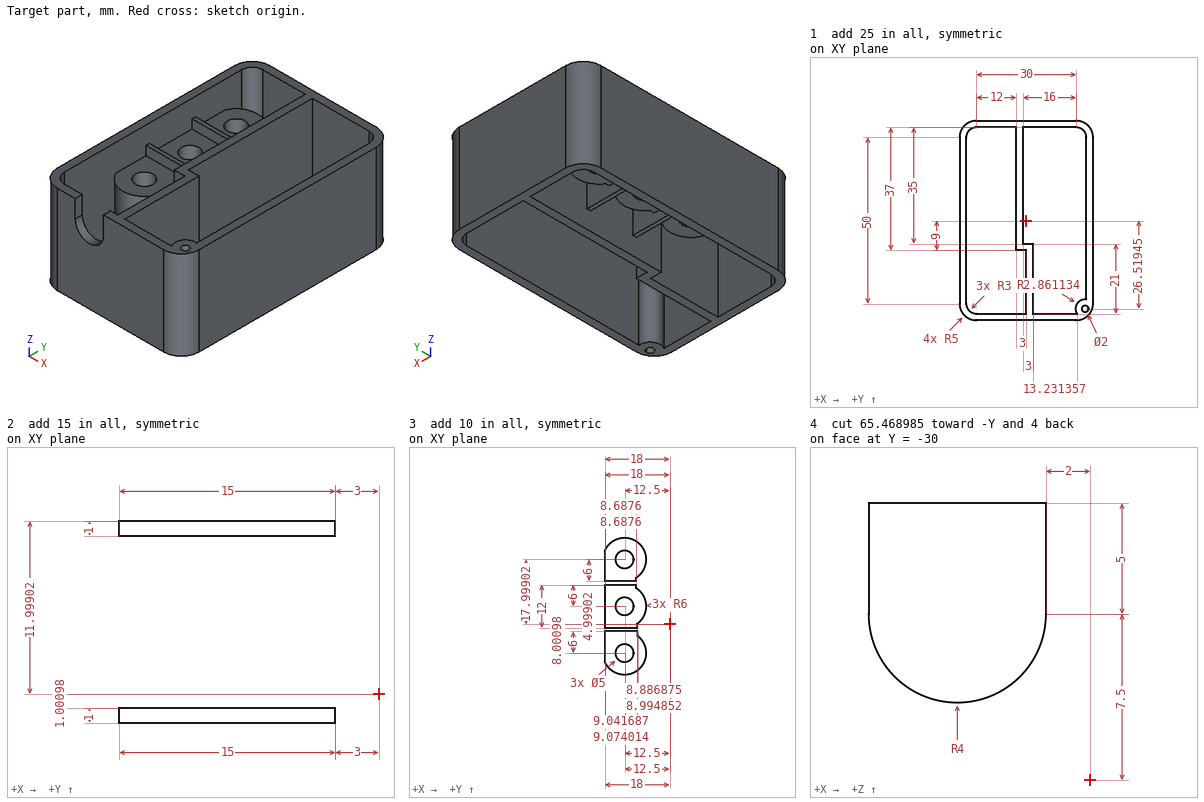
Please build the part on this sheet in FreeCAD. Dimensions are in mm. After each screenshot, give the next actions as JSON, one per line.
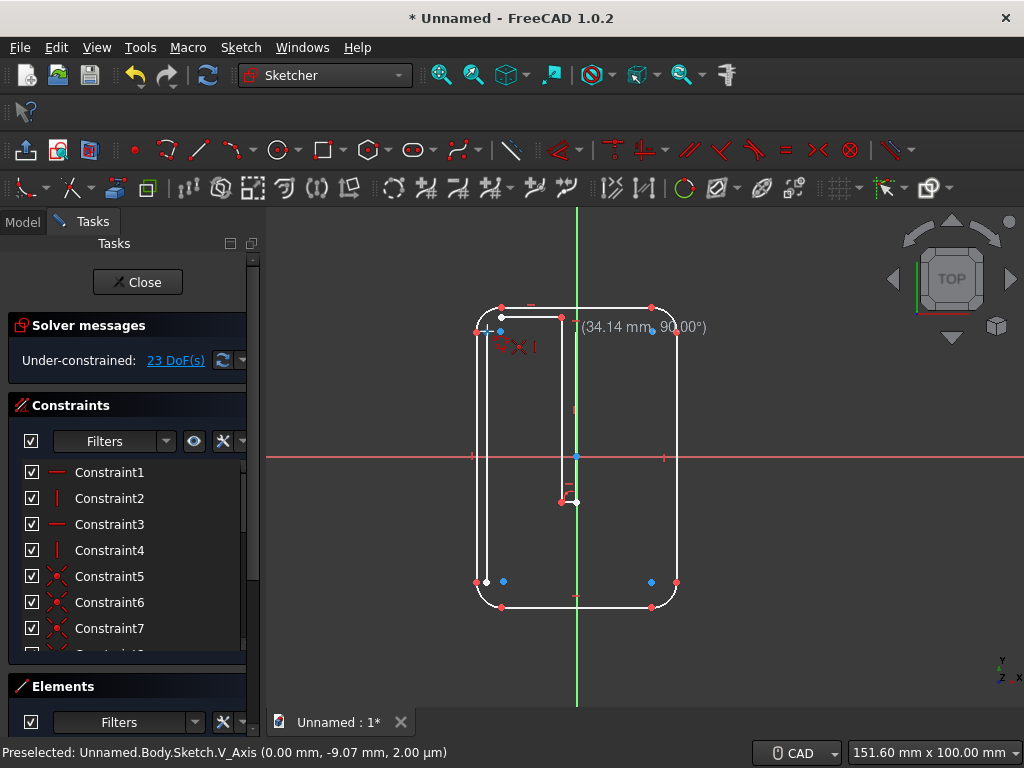
{"action": "scroll", "coordinate": [577, 597], "scroll_direction": "up", "scroll_amount": 3}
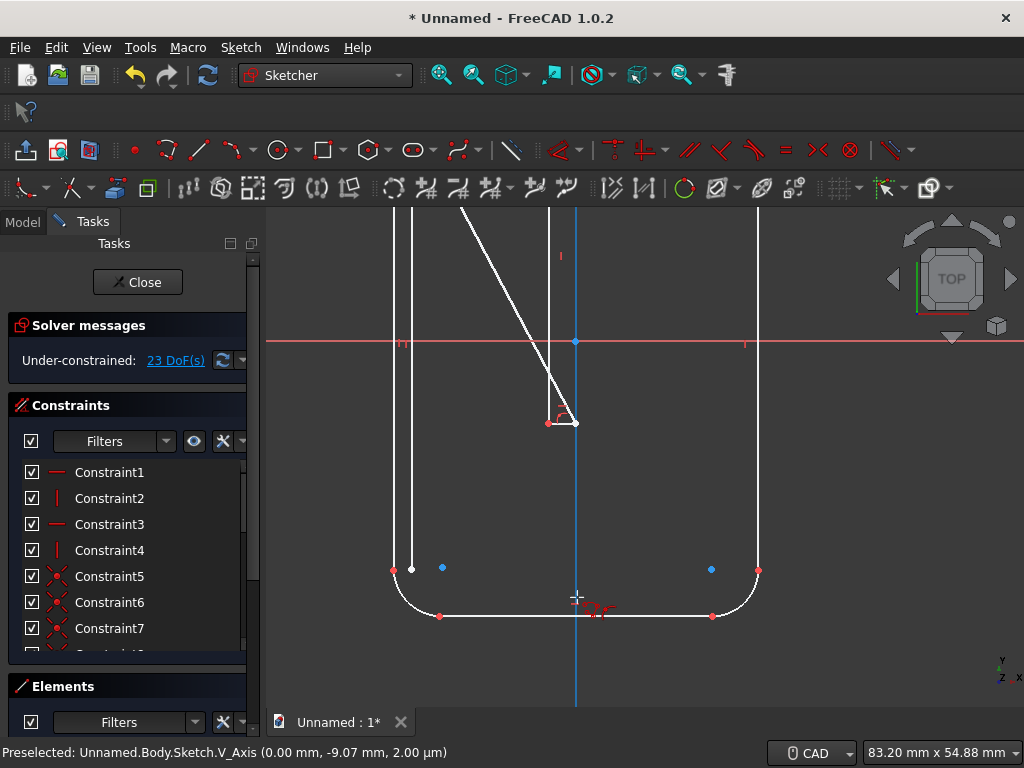
{"action": "left_click", "coordinate": [585, 596]}
{"action": "left_click", "coordinate": [439, 596]}
{"action": "right_click", "coordinate": [439, 596]}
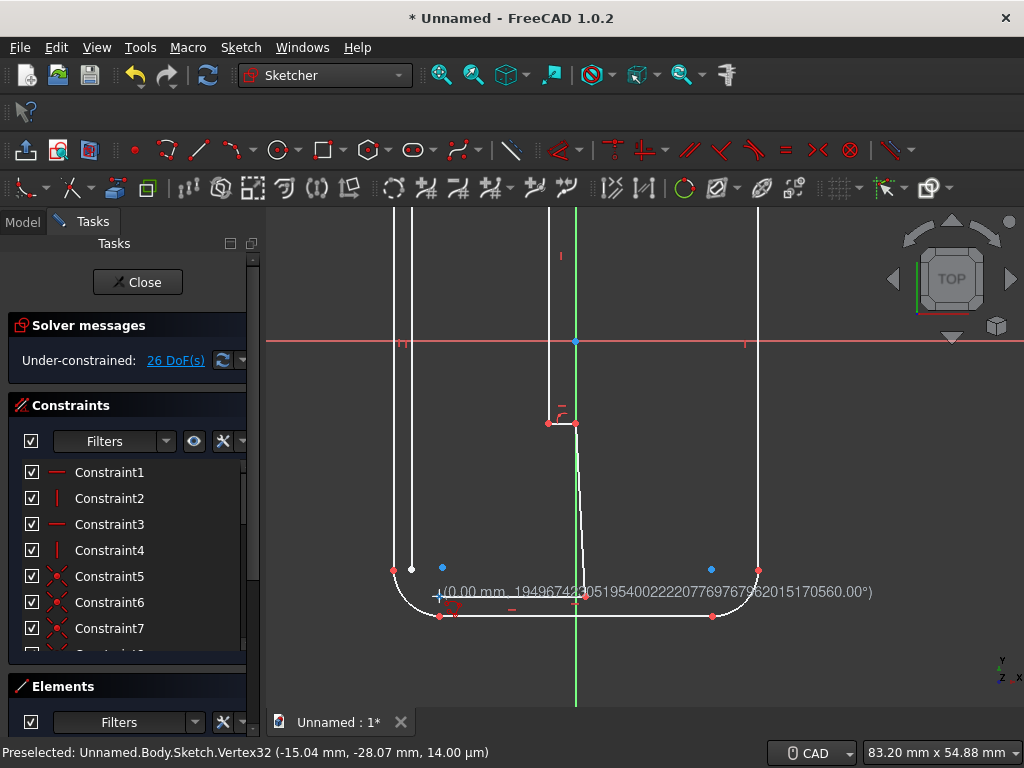
{"action": "left_click", "coordinate": [232, 150]}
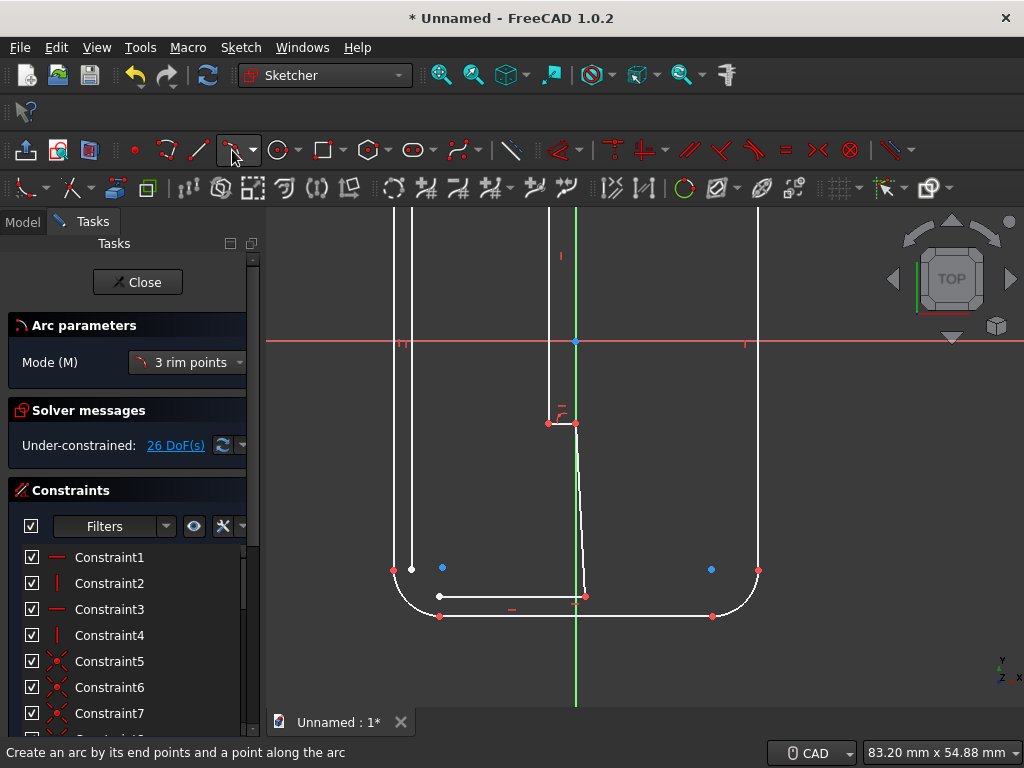
{"action": "scroll", "coordinate": [577, 598], "scroll_direction": "down", "scroll_amount": 3}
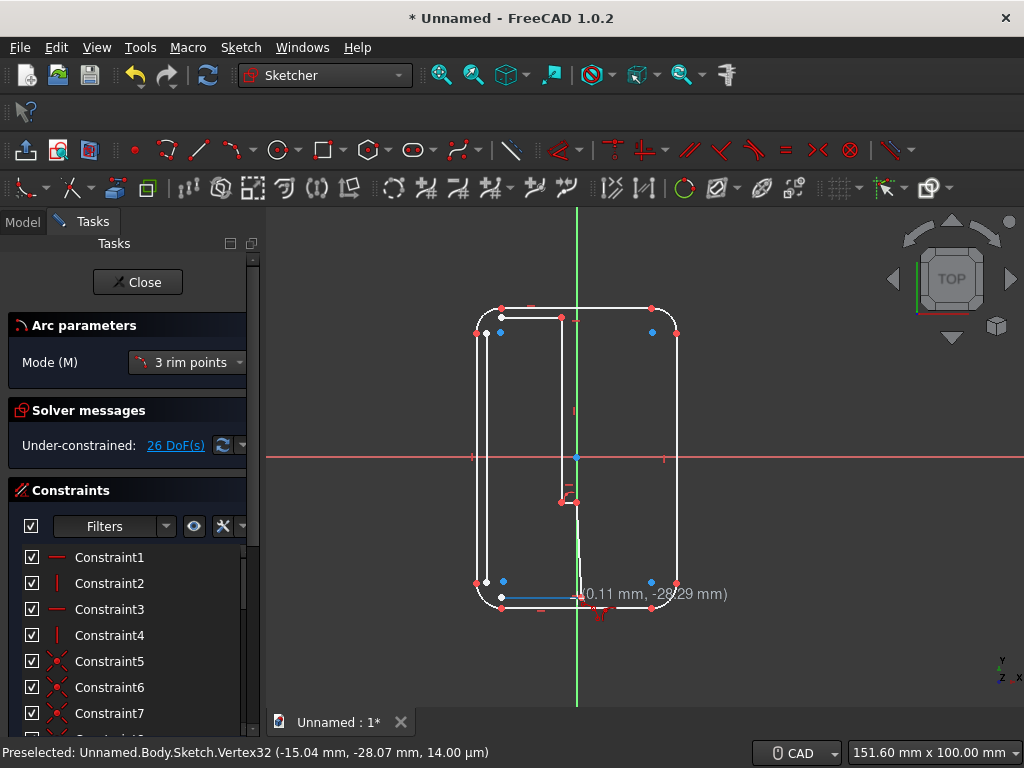
{"action": "scroll", "coordinate": [487, 332], "scroll_direction": "up", "scroll_amount": 3}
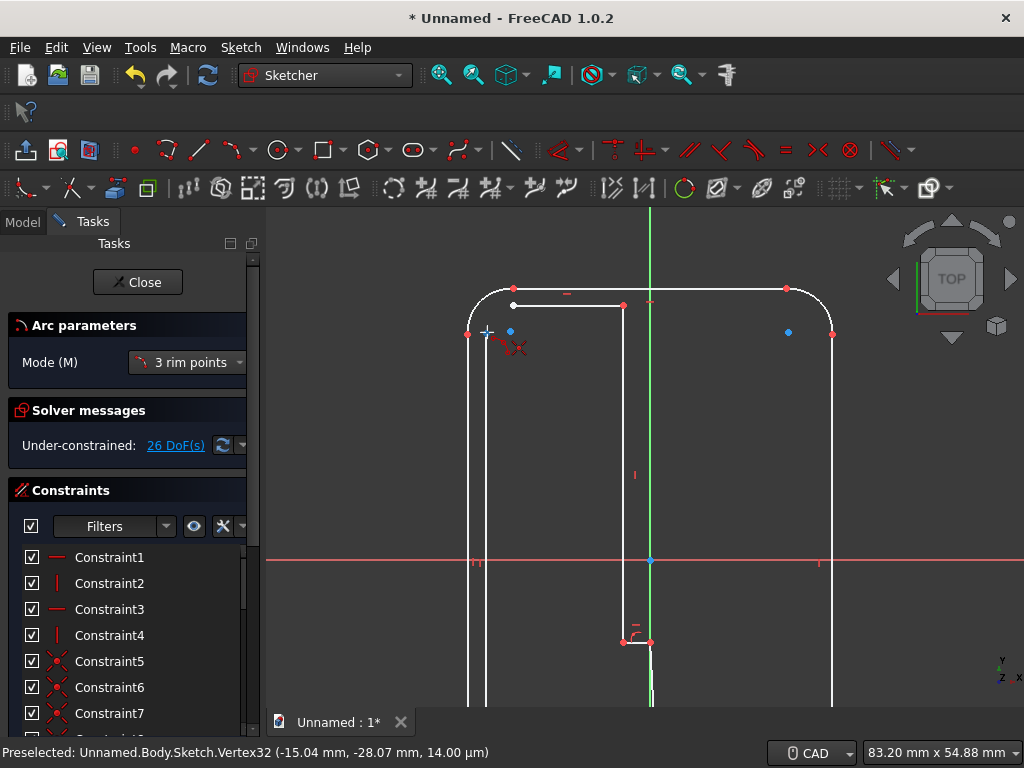
{"action": "left_click", "coordinate": [486, 334]}
{"action": "left_click", "coordinate": [513, 306]}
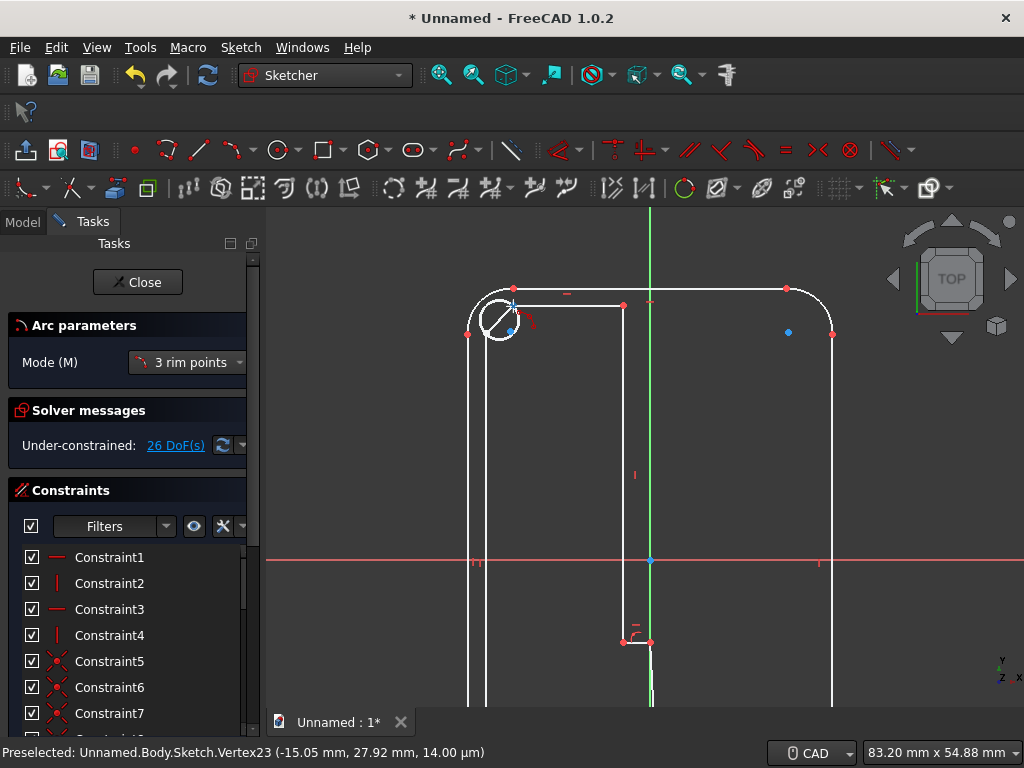
{"action": "scroll", "coordinate": [494, 313], "scroll_direction": "up", "scroll_amount": 4}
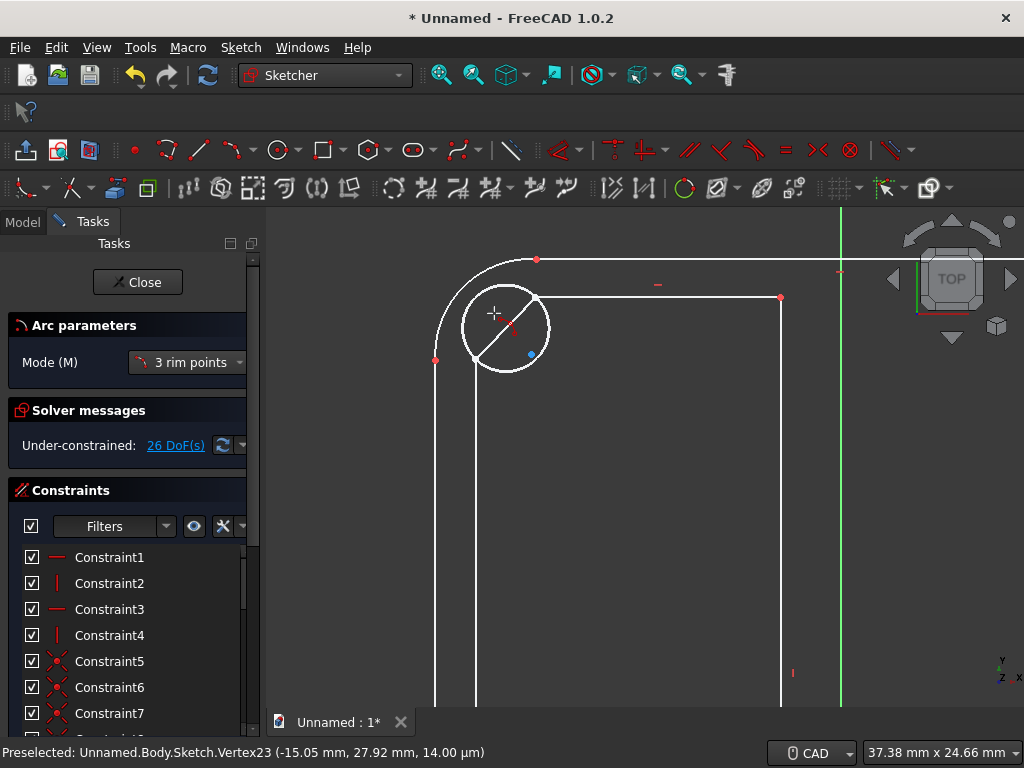
{"action": "left_click", "coordinate": [494, 313]}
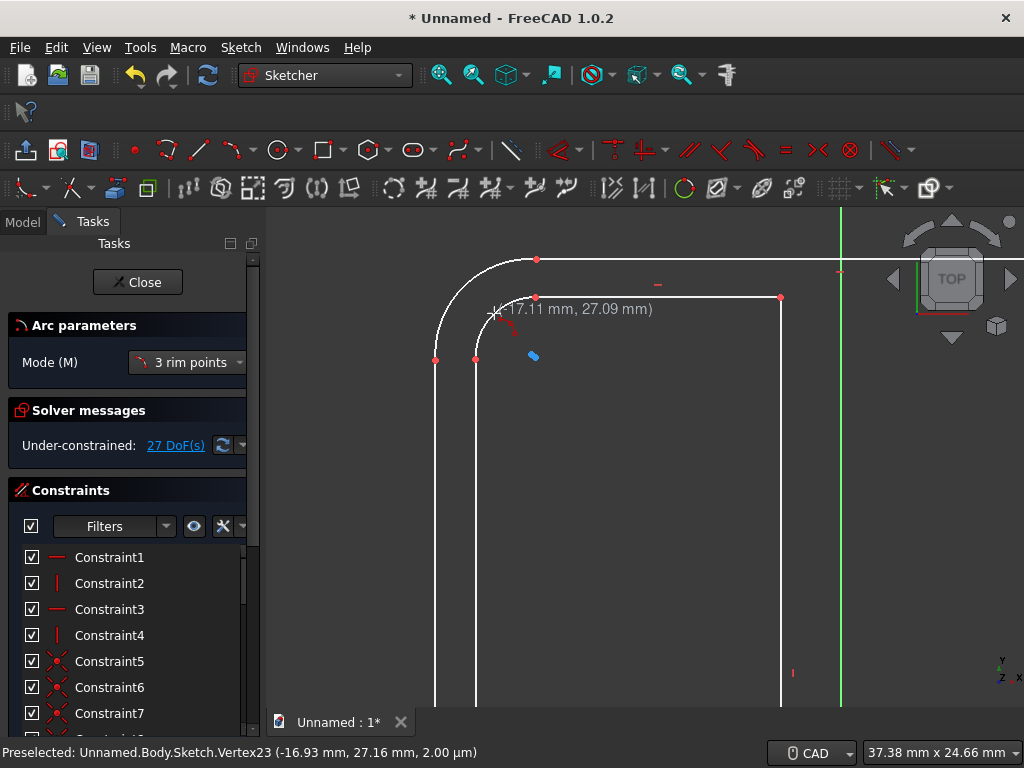
{"action": "scroll", "coordinate": [490, 324], "scroll_direction": "down", "scroll_amount": 7}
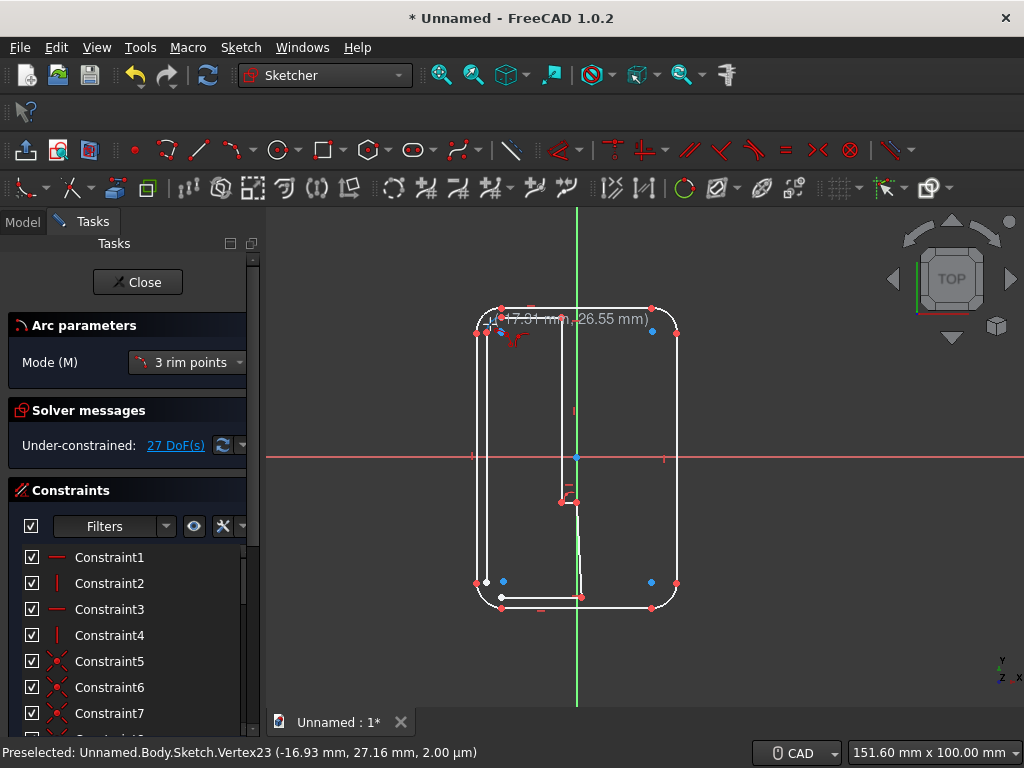
{"action": "scroll", "coordinate": [502, 597], "scroll_direction": "up", "scroll_amount": 3}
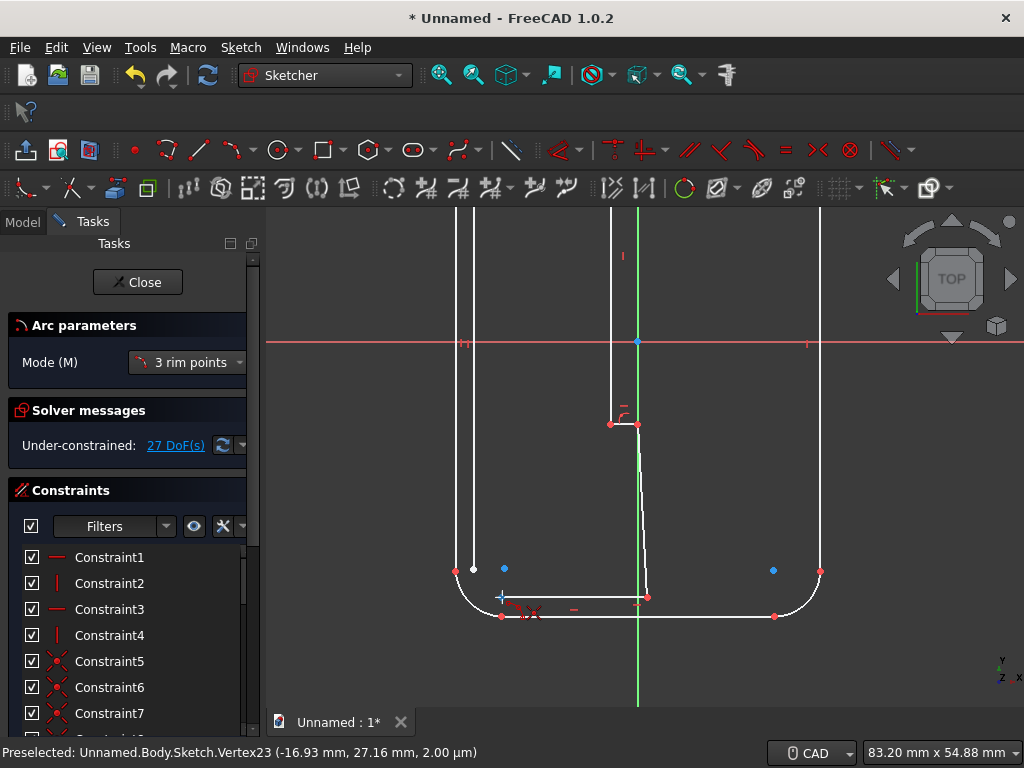
{"action": "left_click", "coordinate": [501, 597]}
{"action": "left_click", "coordinate": [474, 570]}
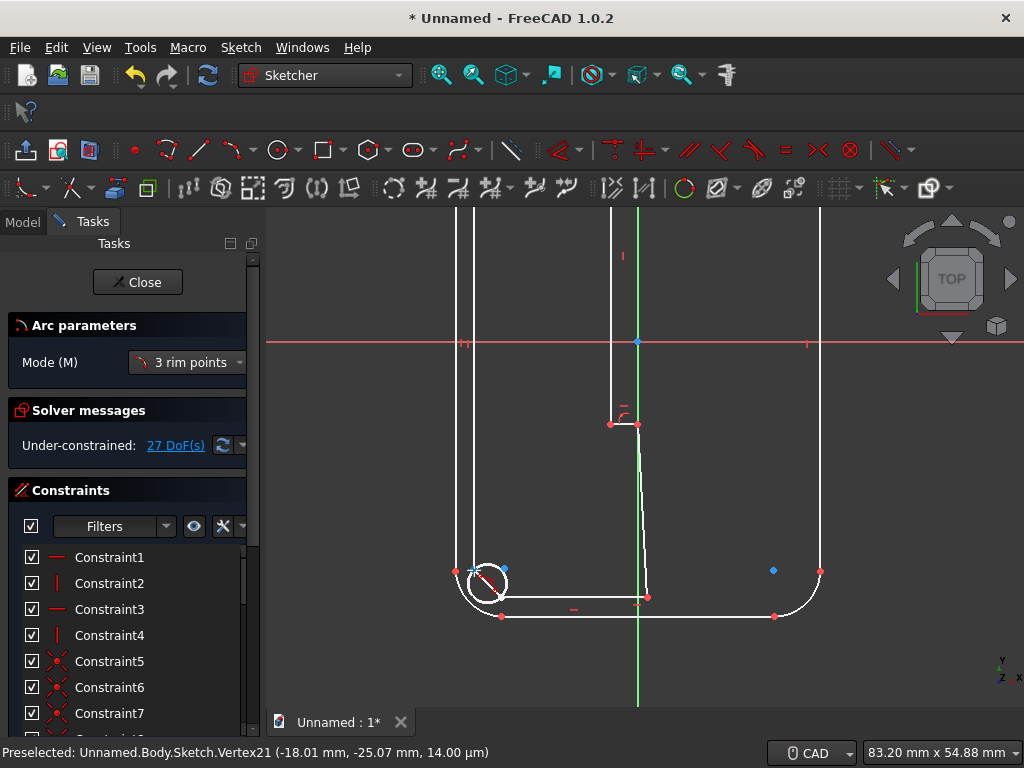
{"action": "scroll", "coordinate": [482, 589], "scroll_direction": "up", "scroll_amount": 4}